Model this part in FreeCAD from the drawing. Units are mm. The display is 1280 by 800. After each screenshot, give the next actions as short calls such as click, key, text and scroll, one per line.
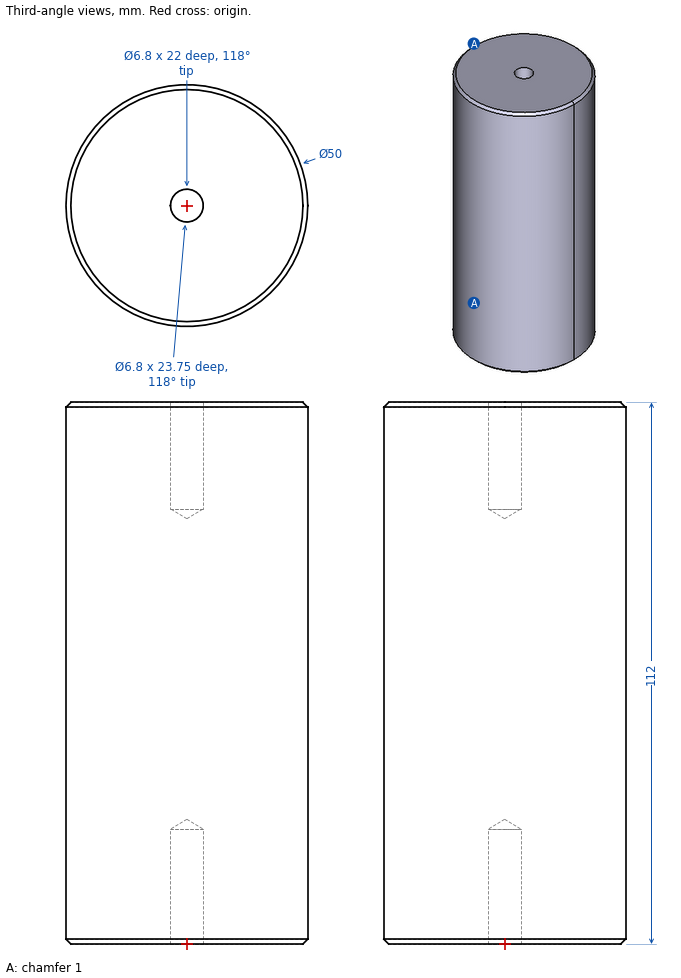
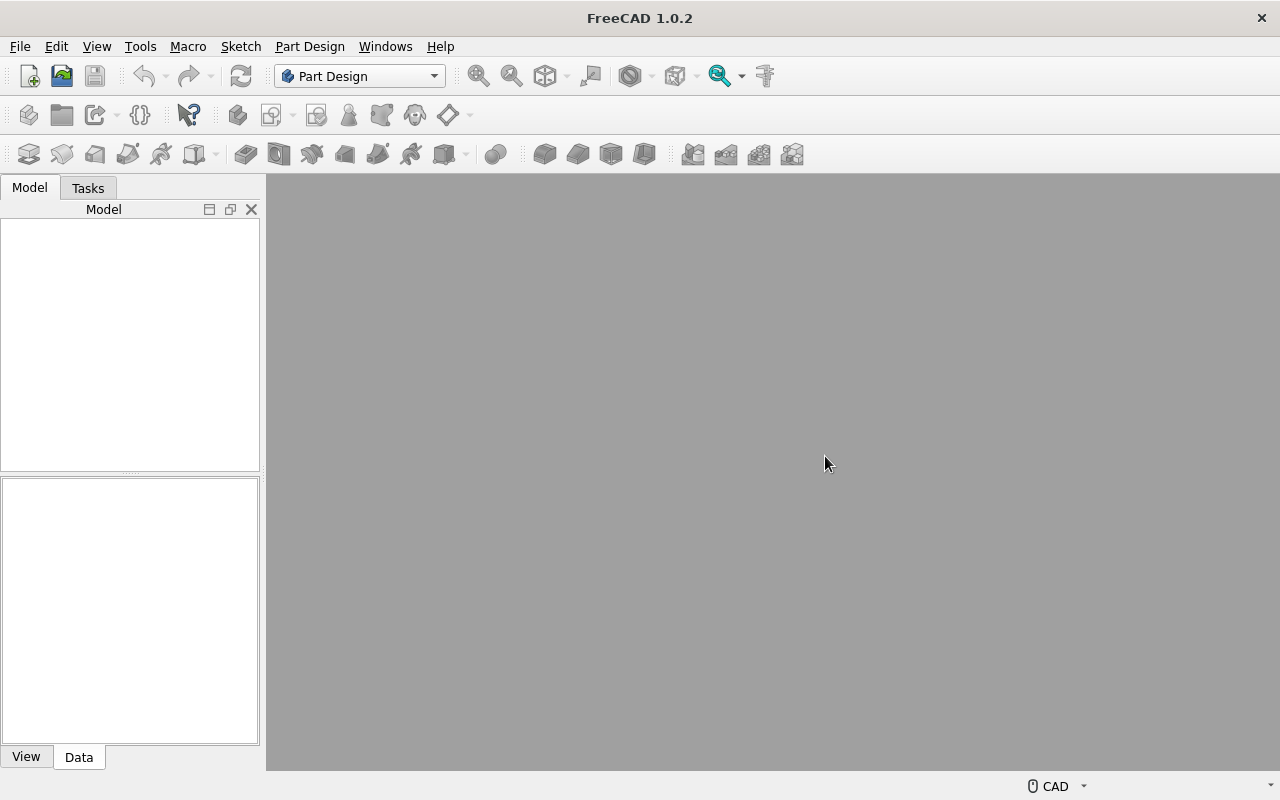
key(ctrl+n)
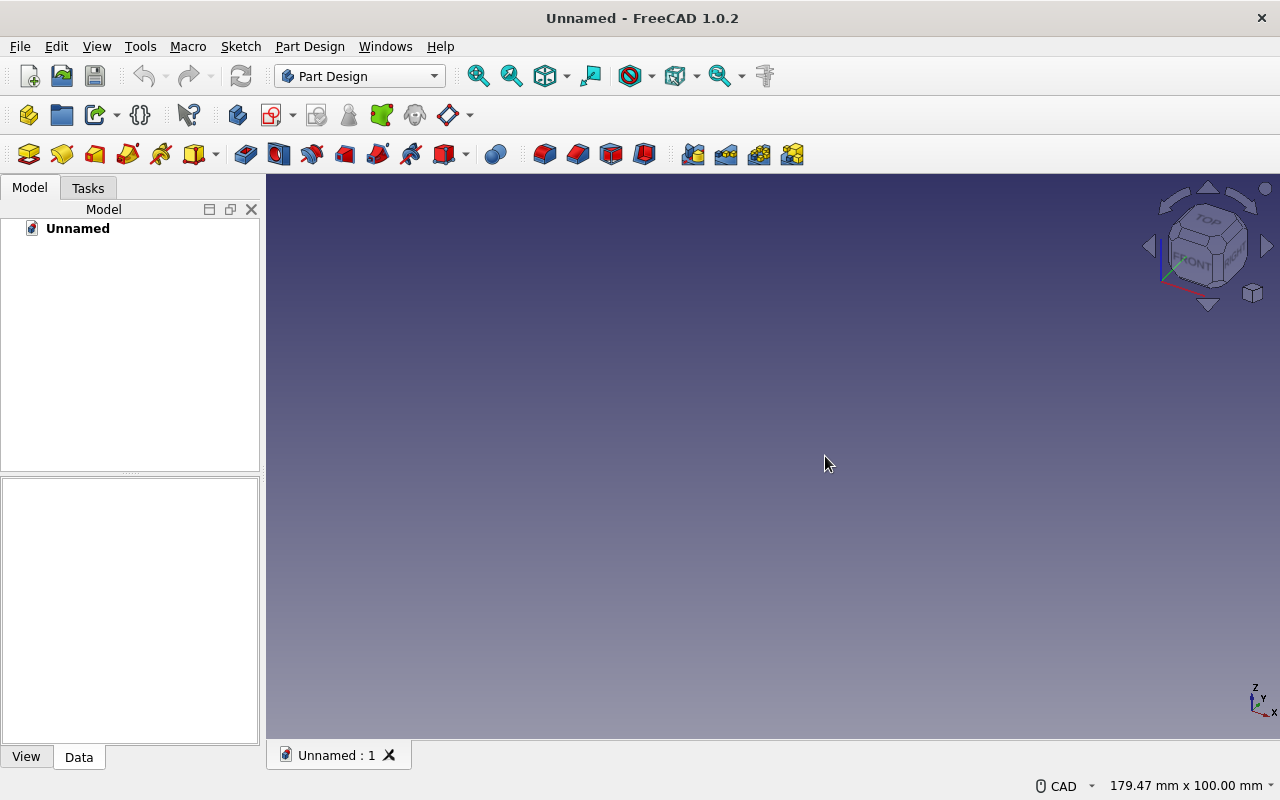
click(270, 116)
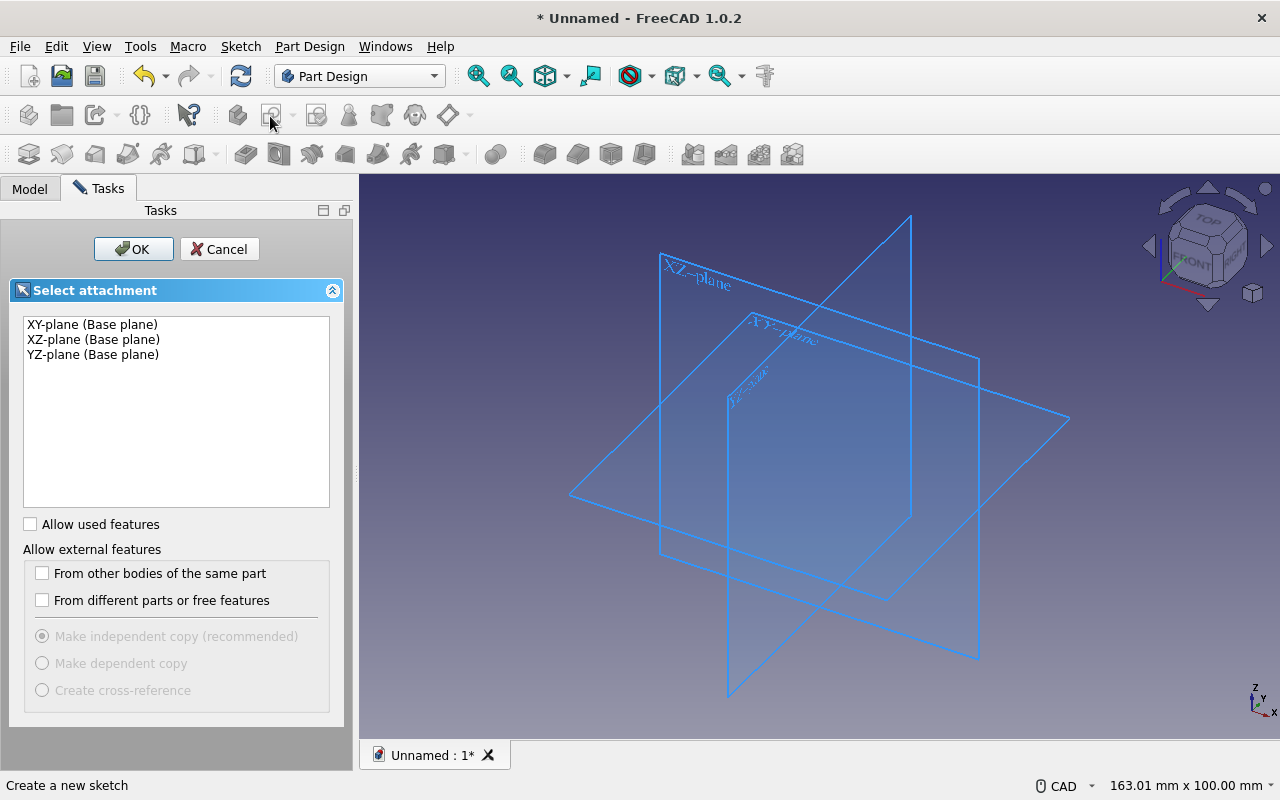
click(84, 324)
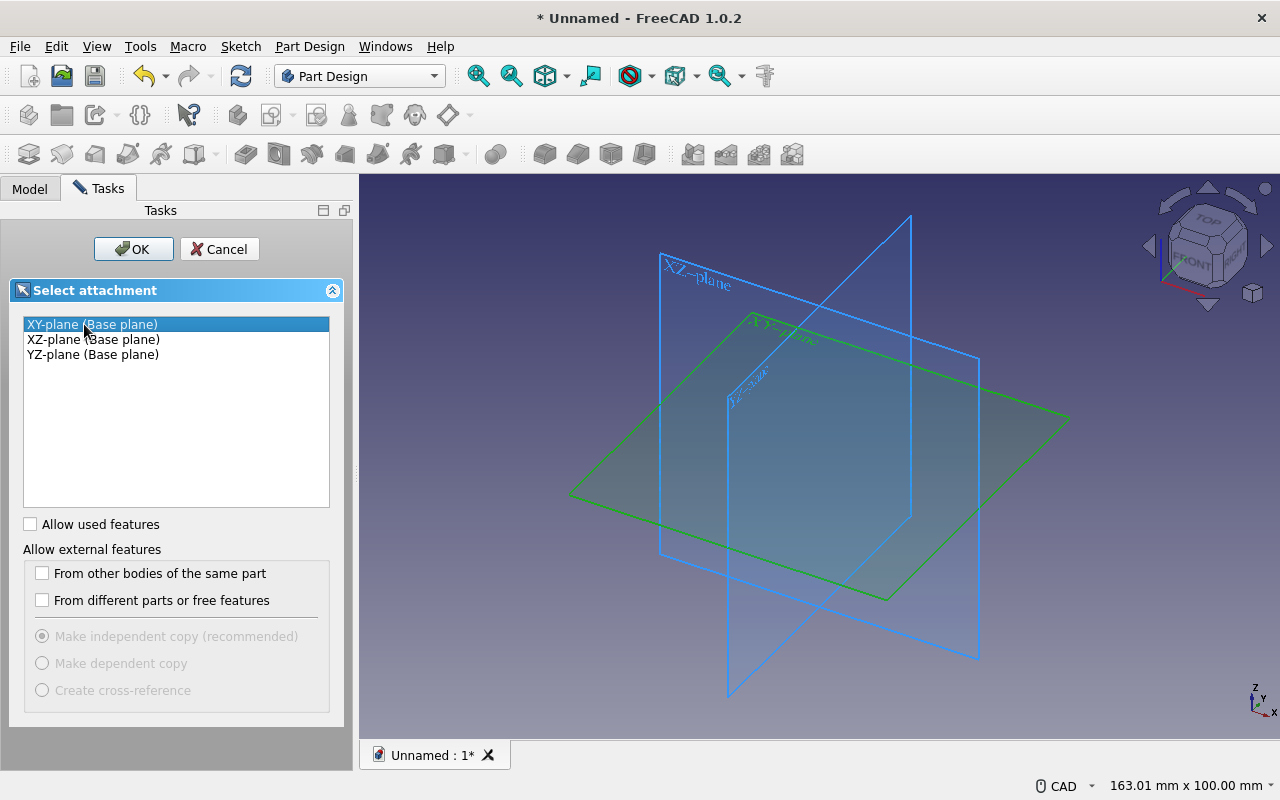
click(134, 249)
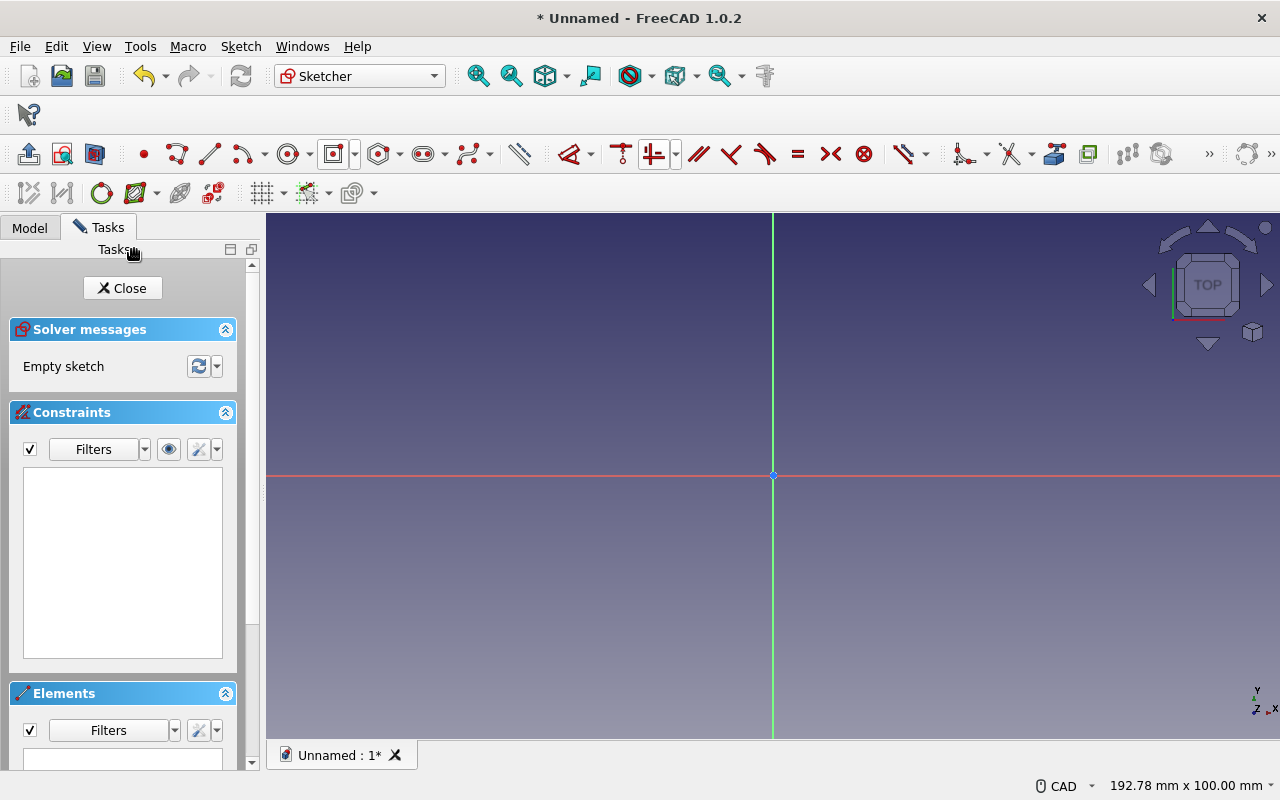
click(288, 154)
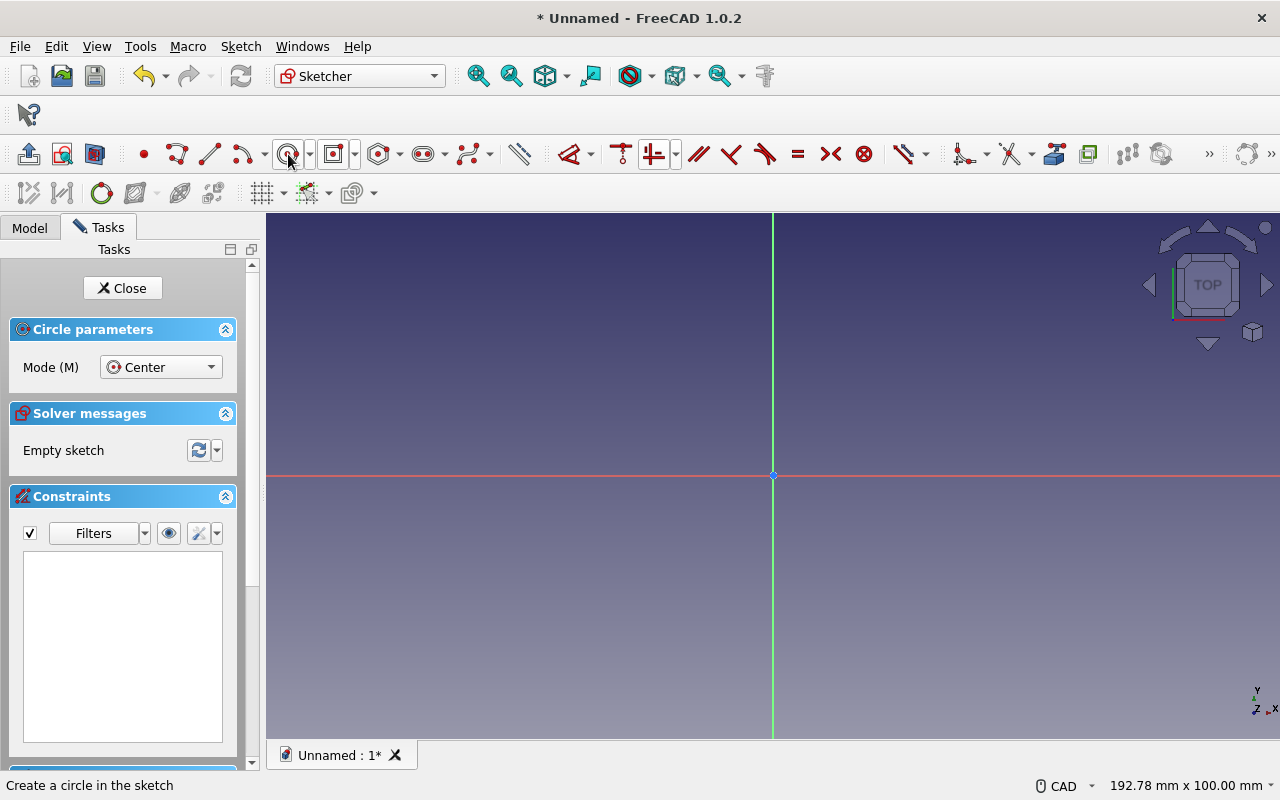
click(773, 476)
click(866, 383)
key(Escape)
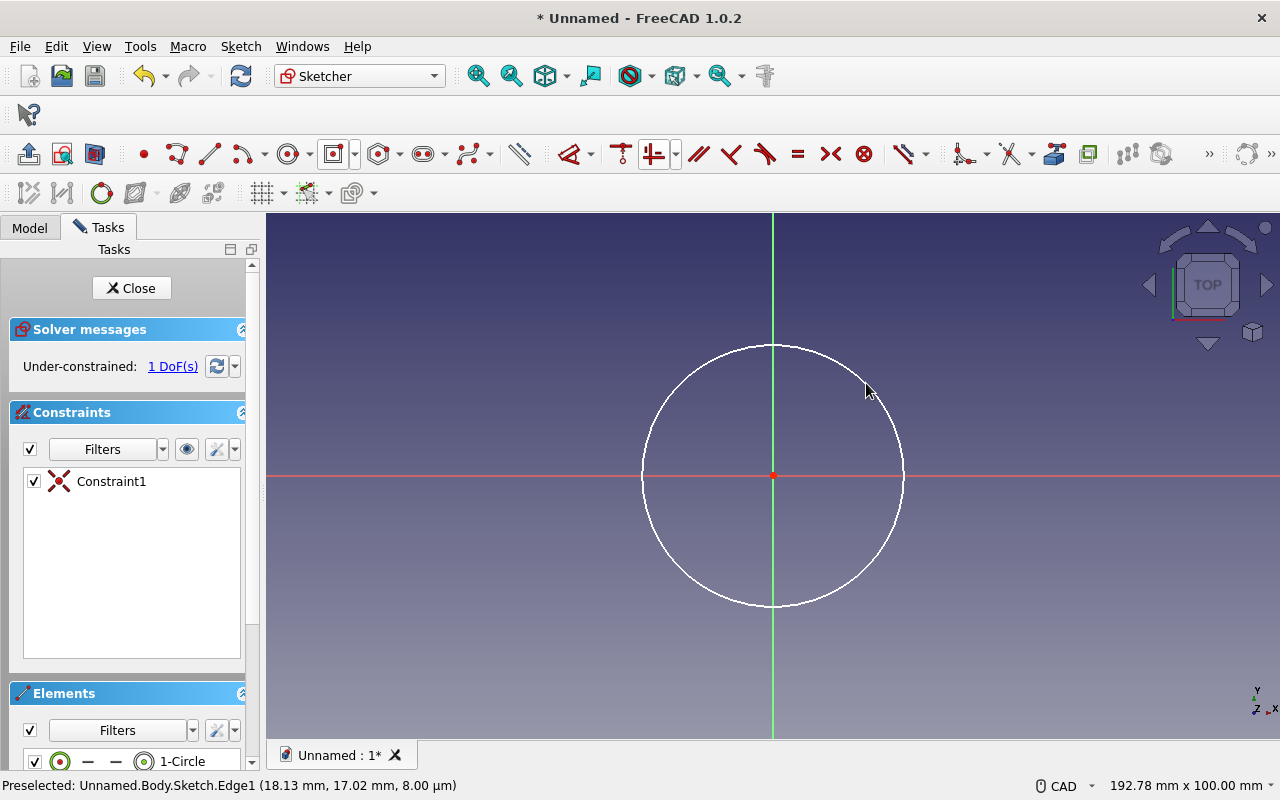
key(d)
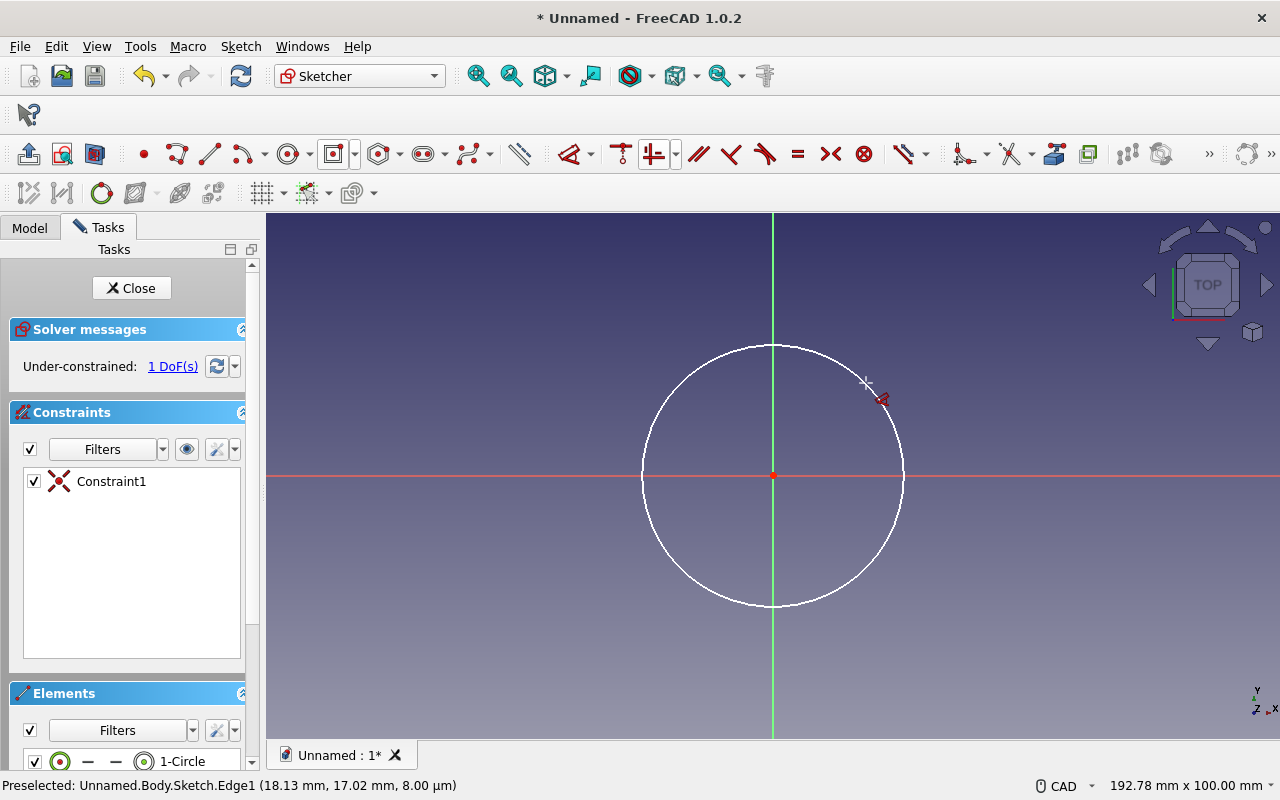
click(865, 383)
click(888, 360)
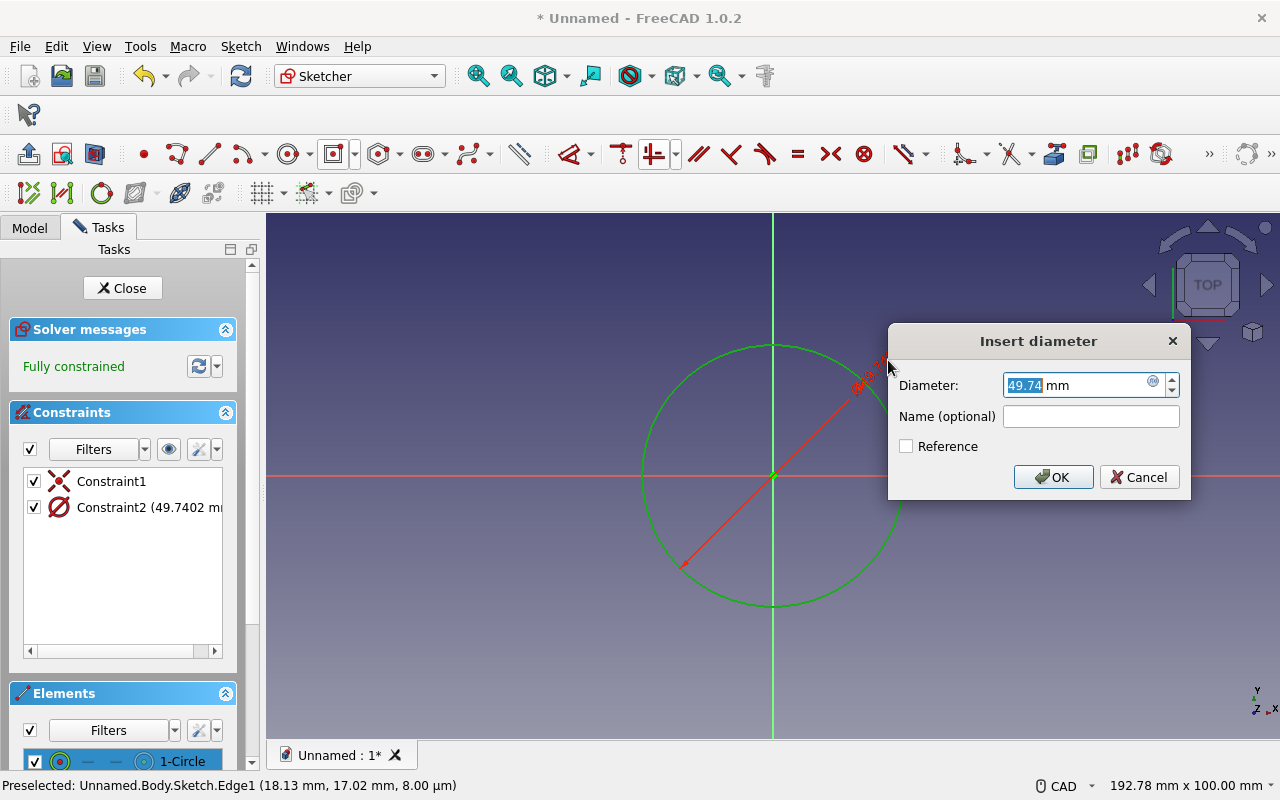
text(50)
key(Return)
key(Escape)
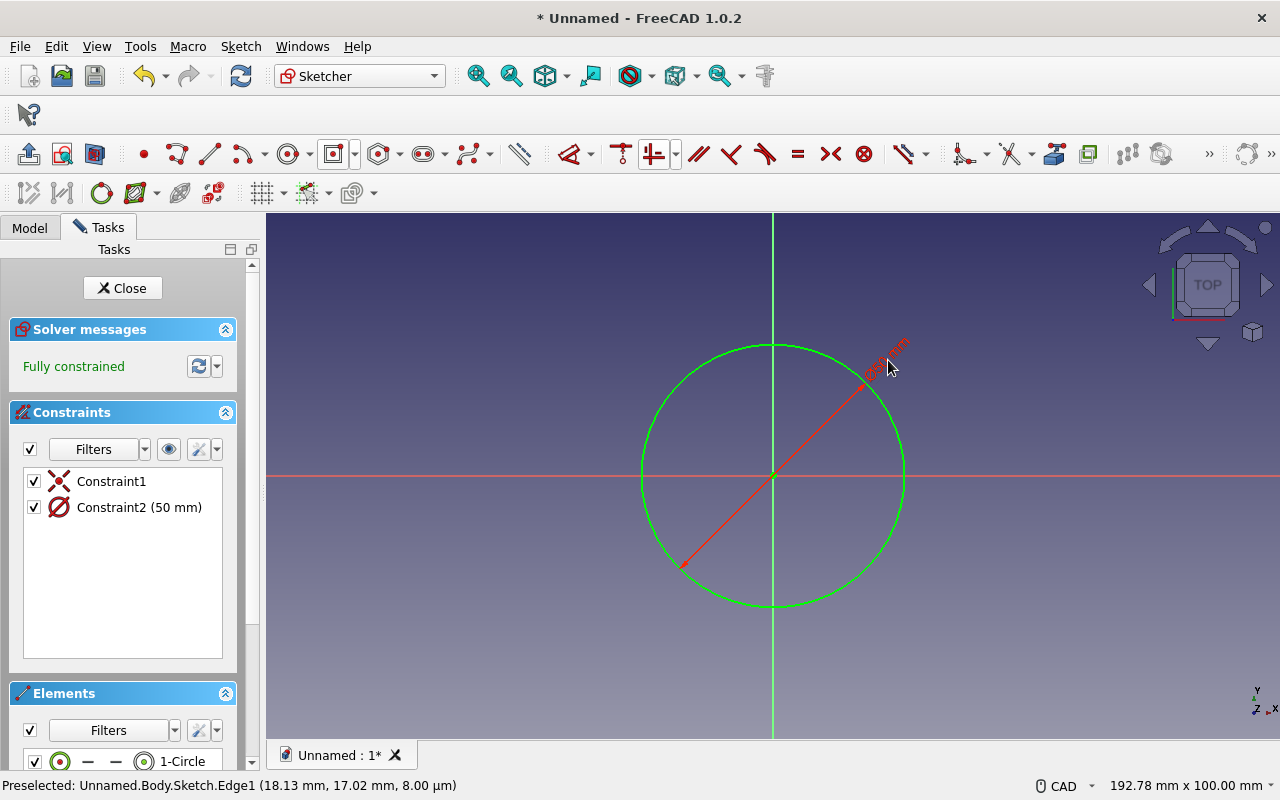
click(123, 288)